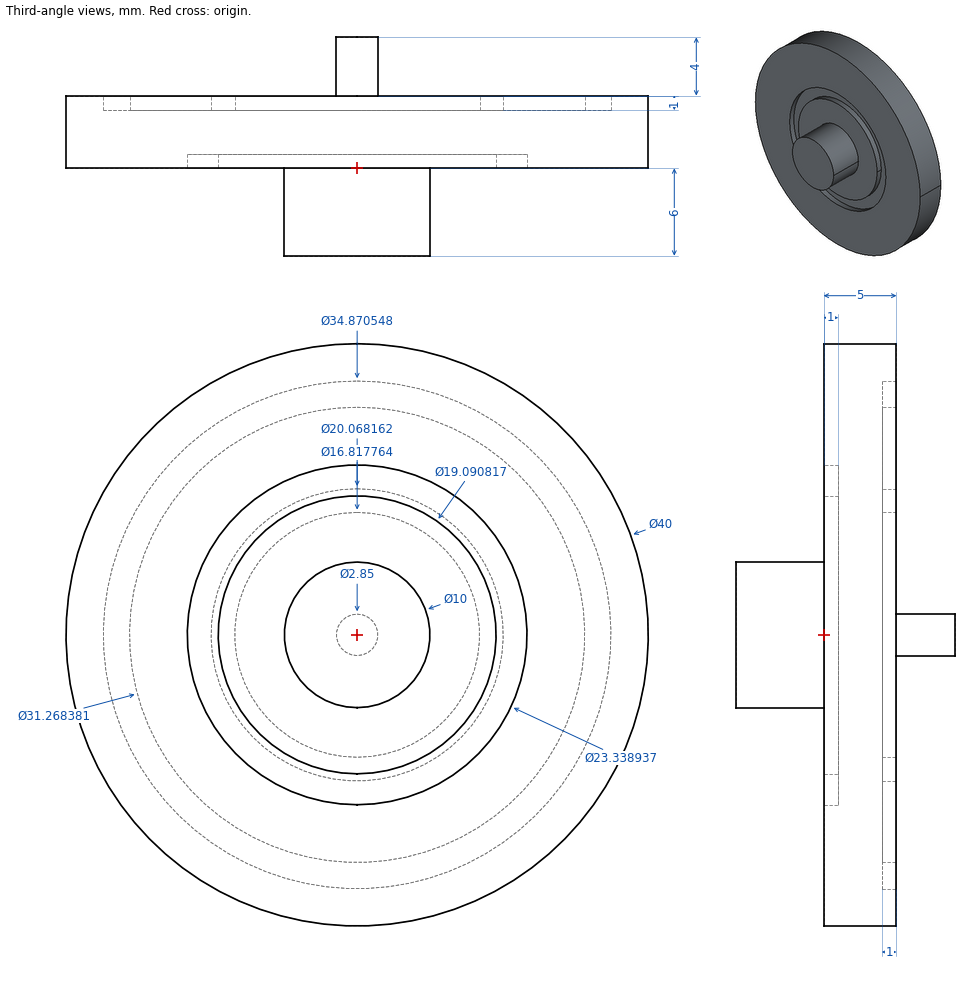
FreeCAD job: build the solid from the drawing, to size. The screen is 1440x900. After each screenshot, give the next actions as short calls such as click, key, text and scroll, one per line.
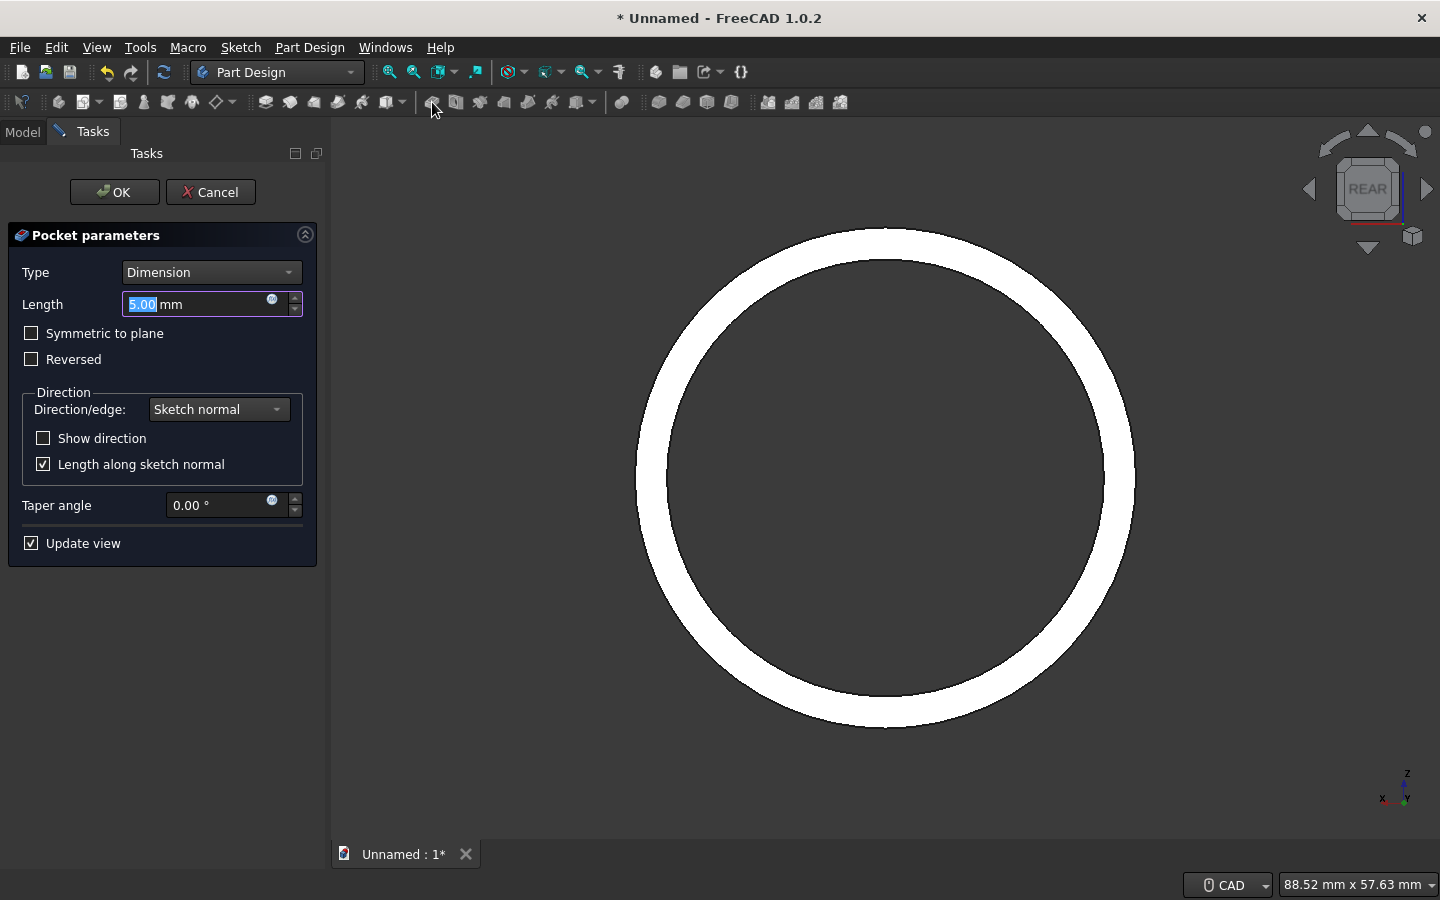
text(1)
key(Tab)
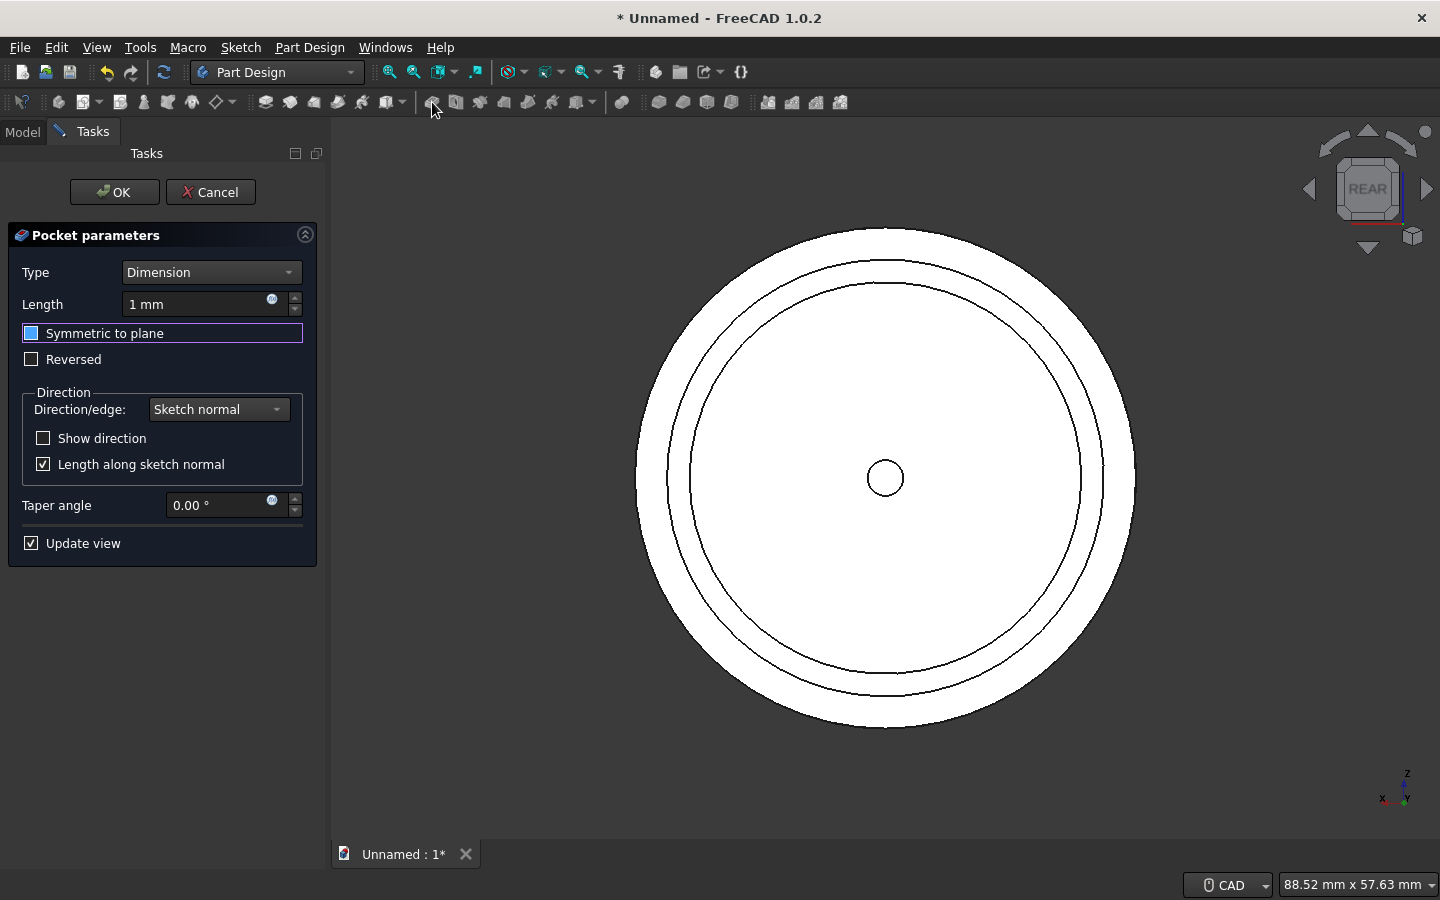
click(115, 192)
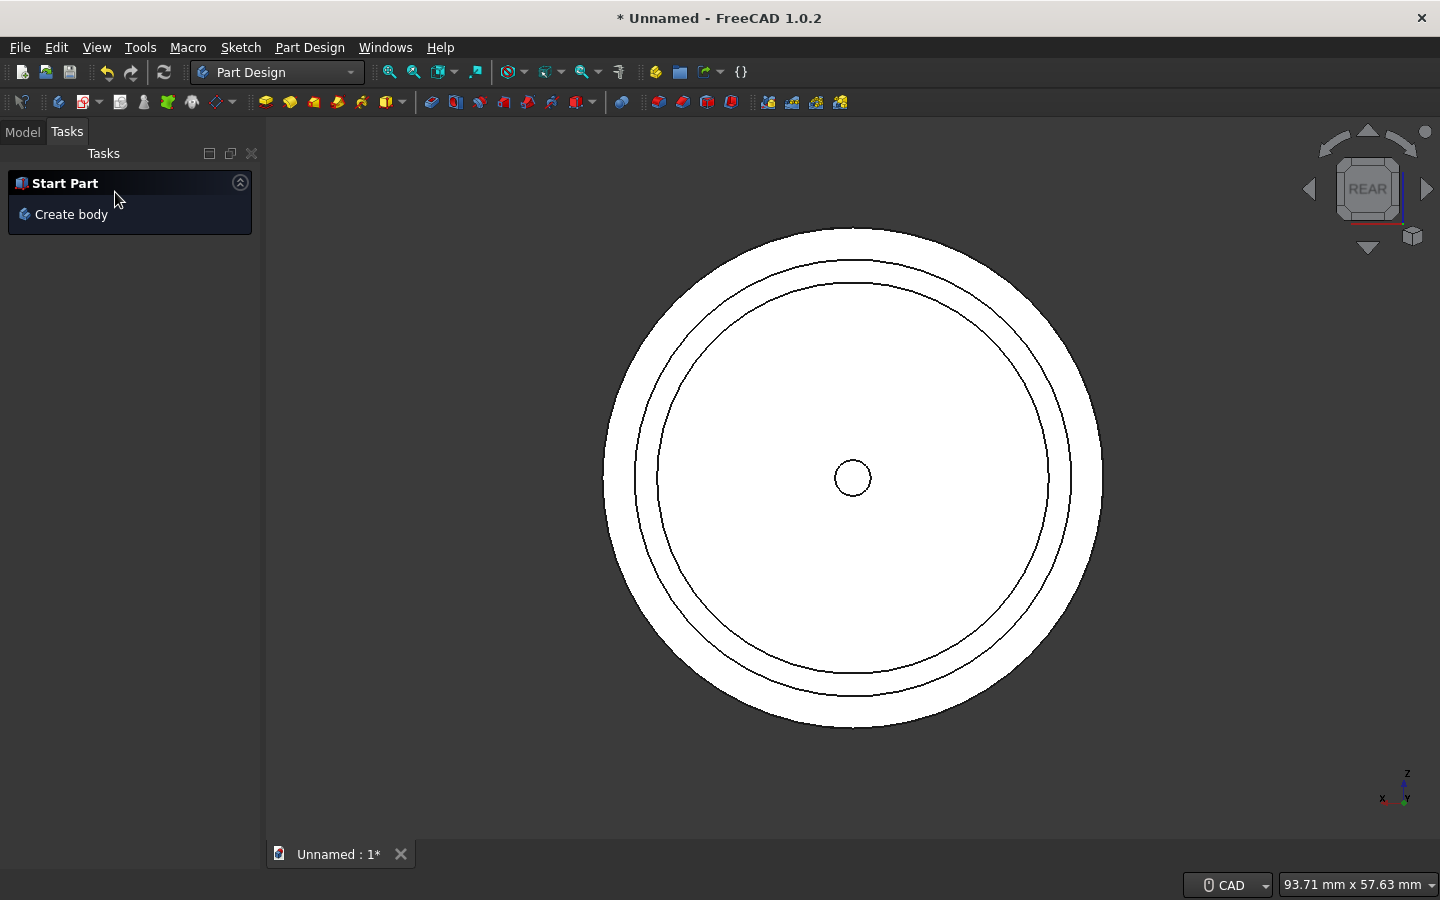
click(741, 477)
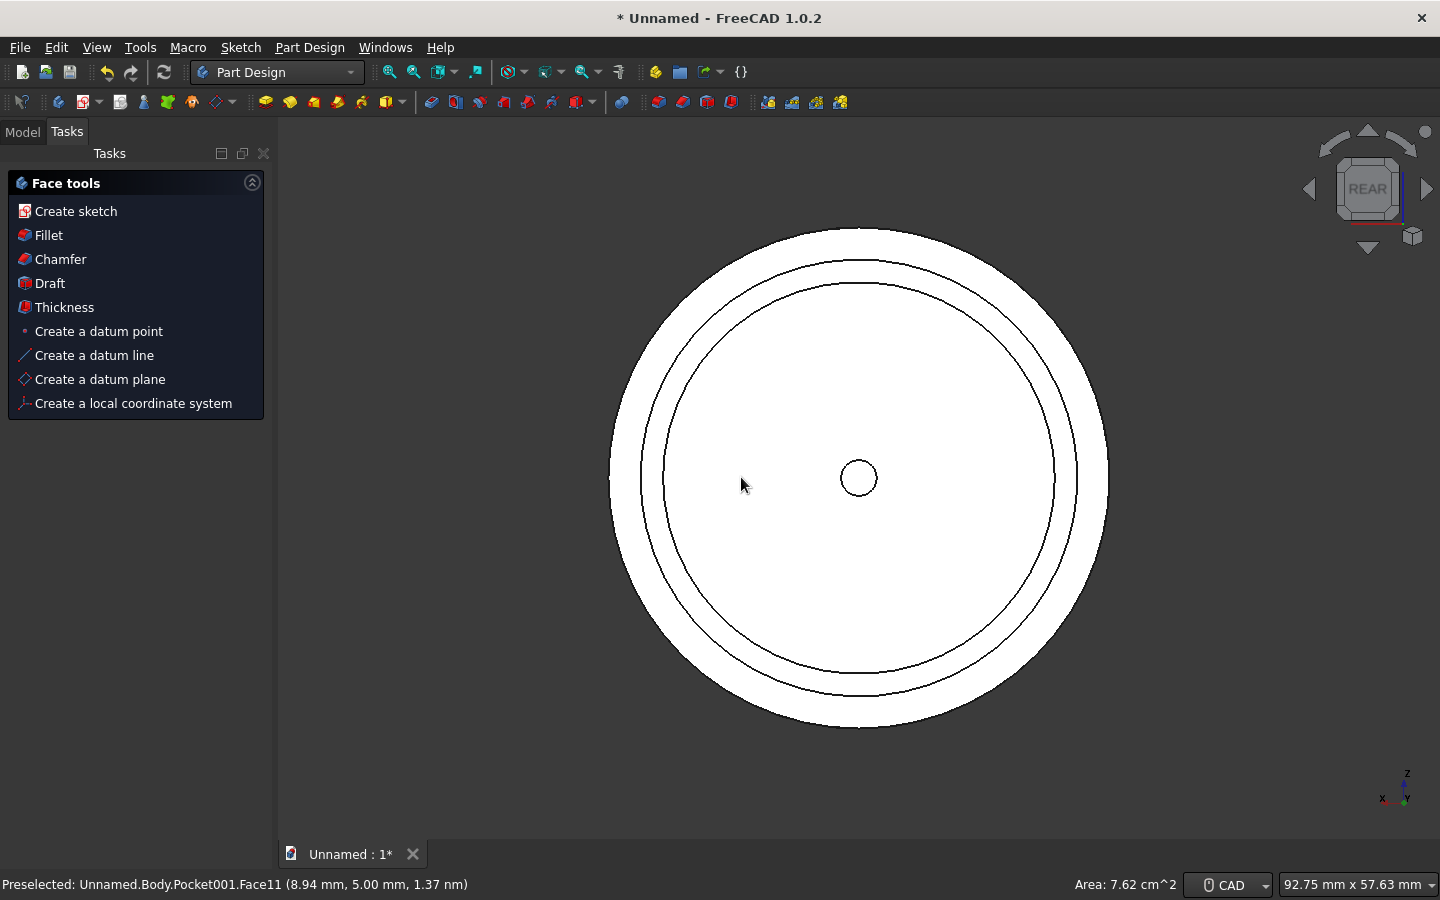
click(84, 102)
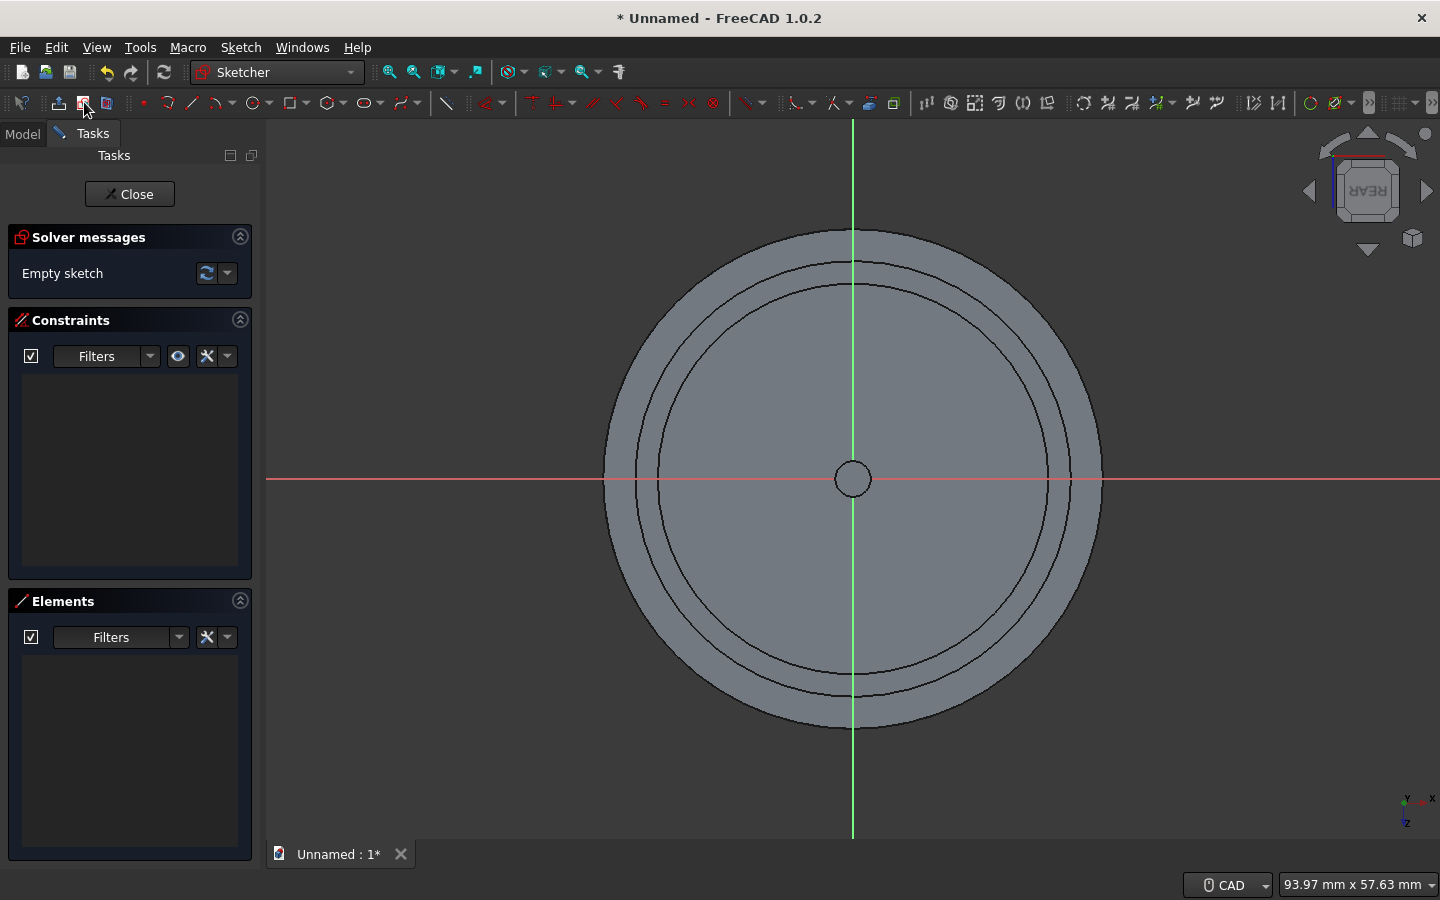
key(q)
key(s)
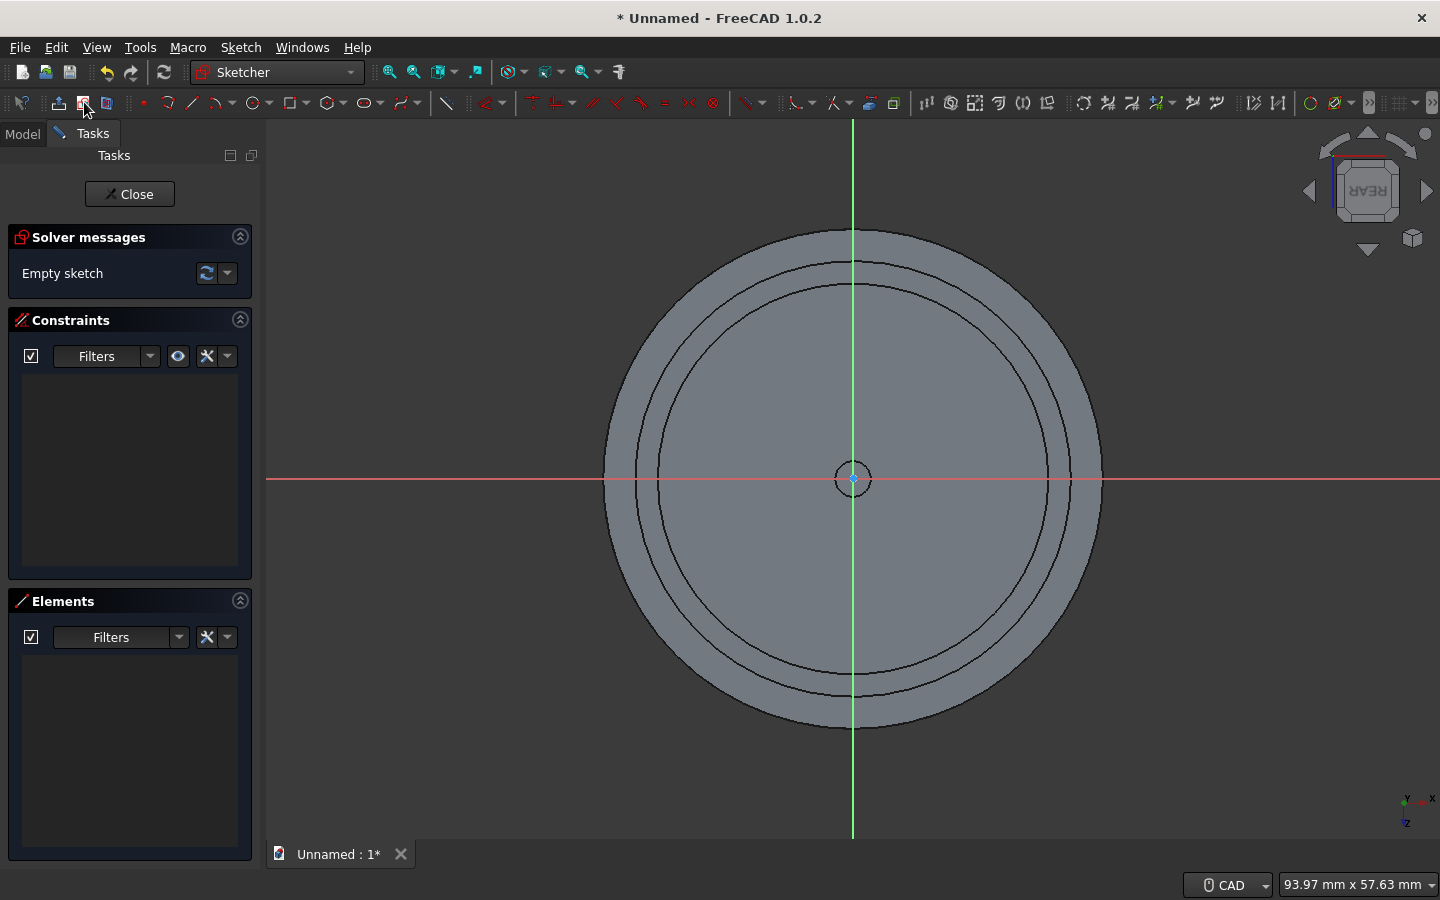
scroll(936, 479, up, 3)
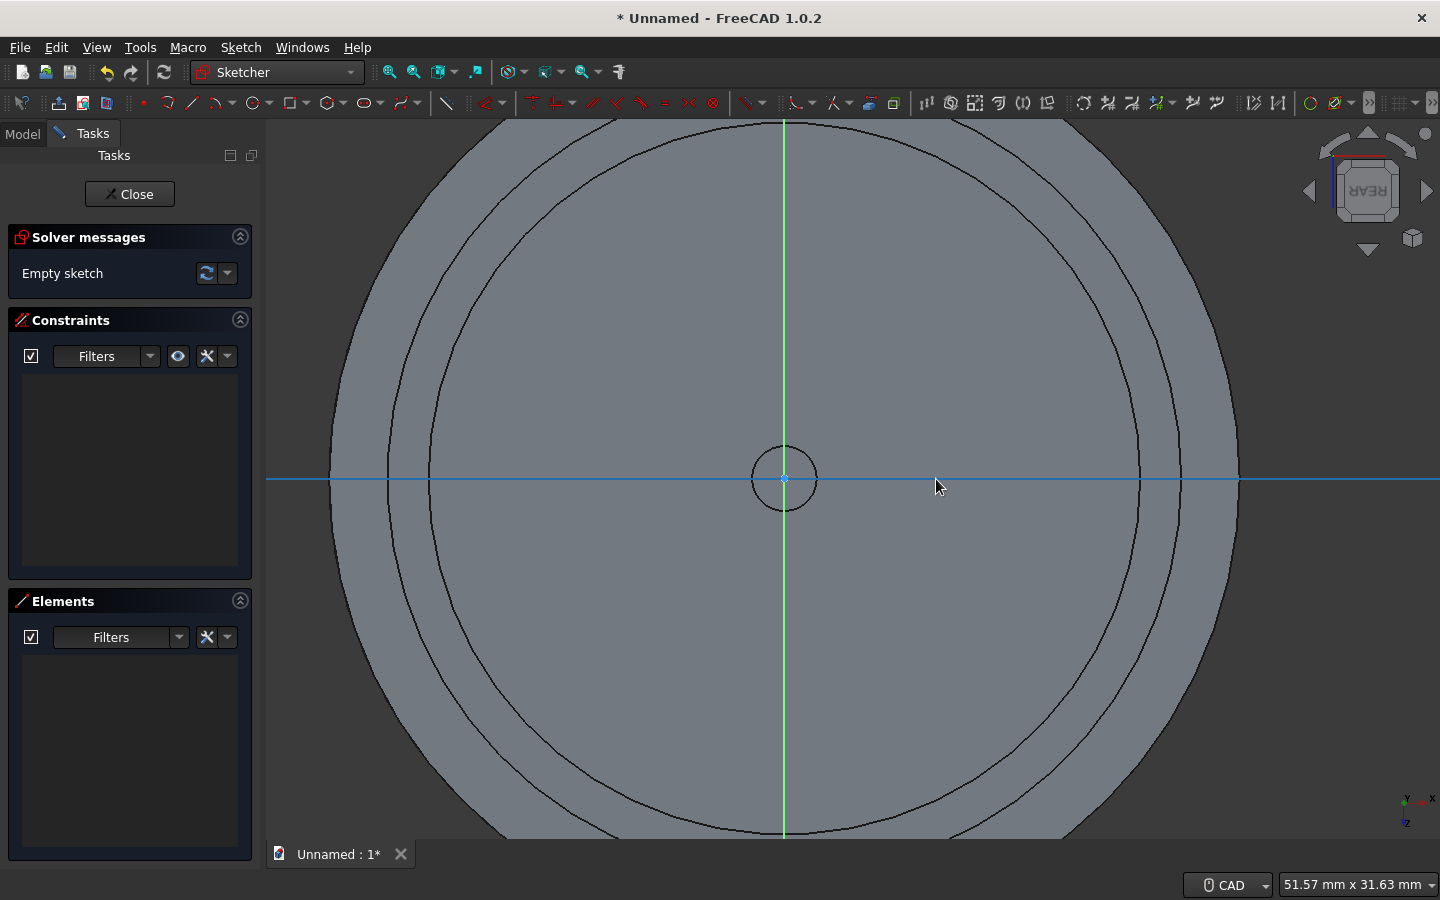
click(254, 104)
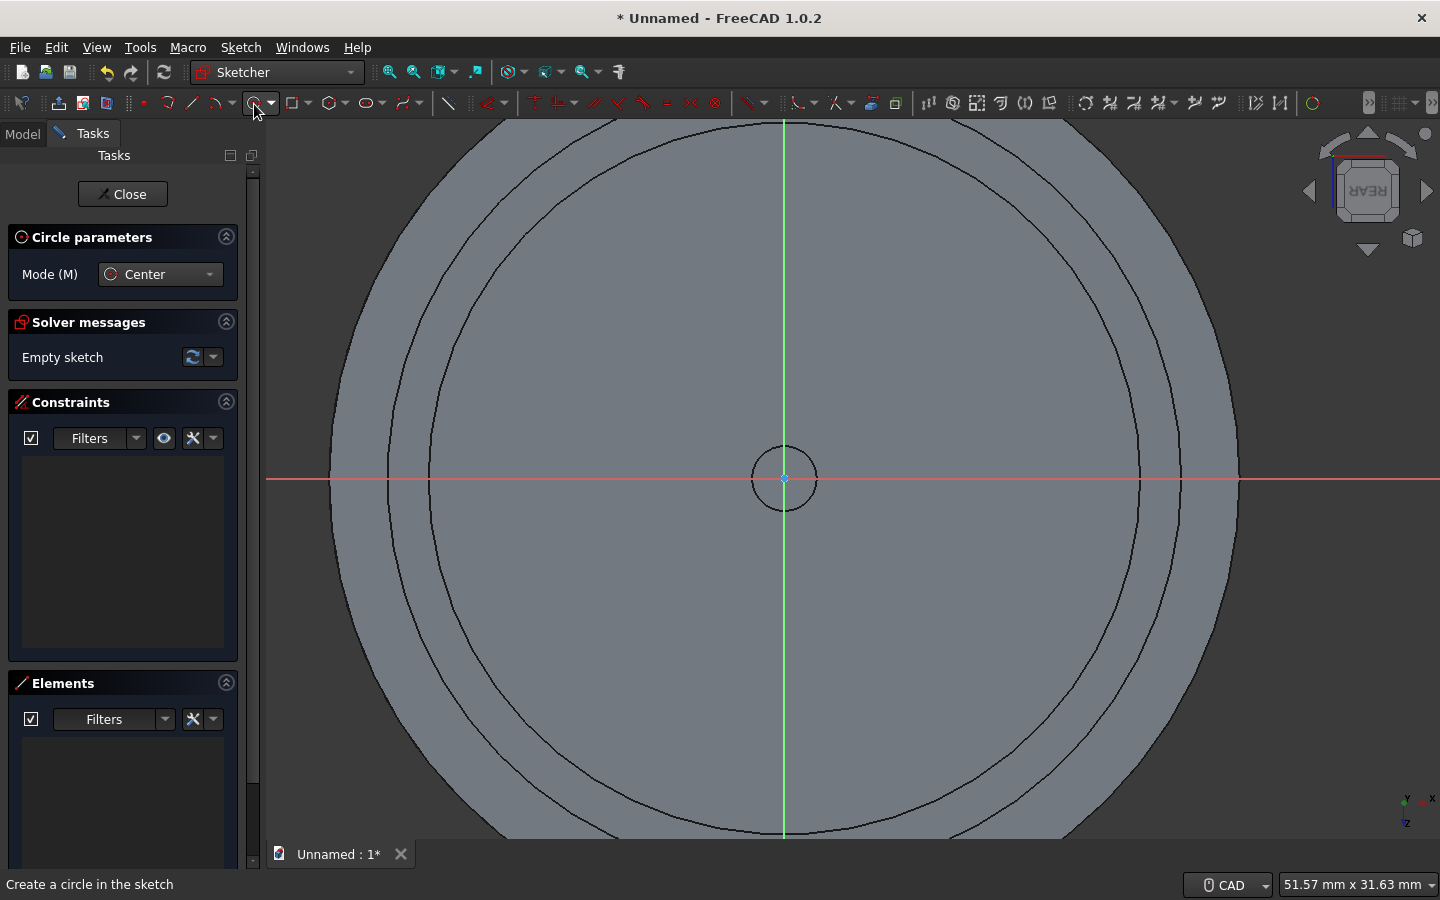
click(784, 479)
click(946, 317)